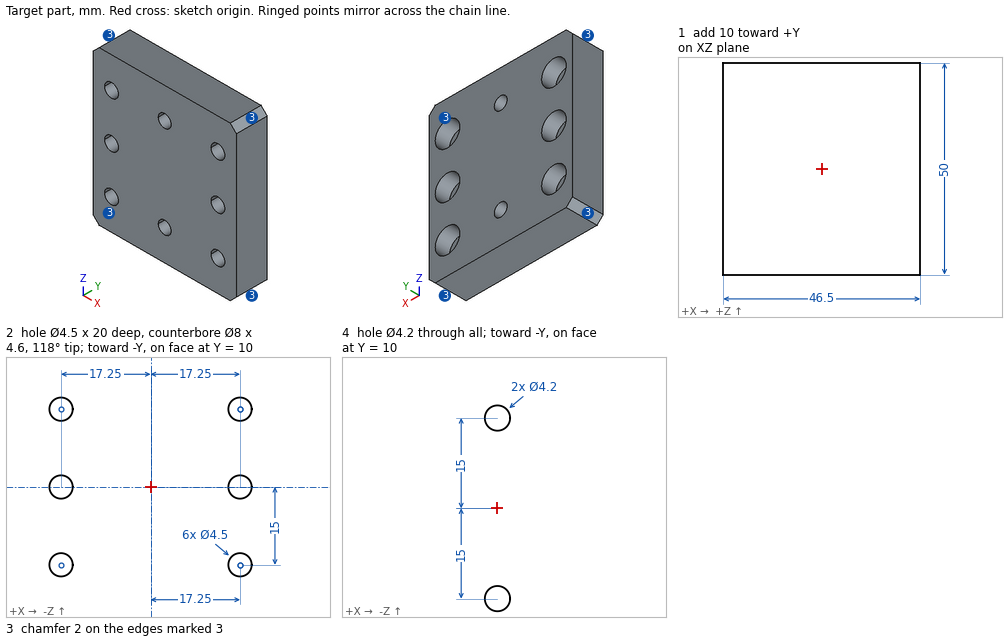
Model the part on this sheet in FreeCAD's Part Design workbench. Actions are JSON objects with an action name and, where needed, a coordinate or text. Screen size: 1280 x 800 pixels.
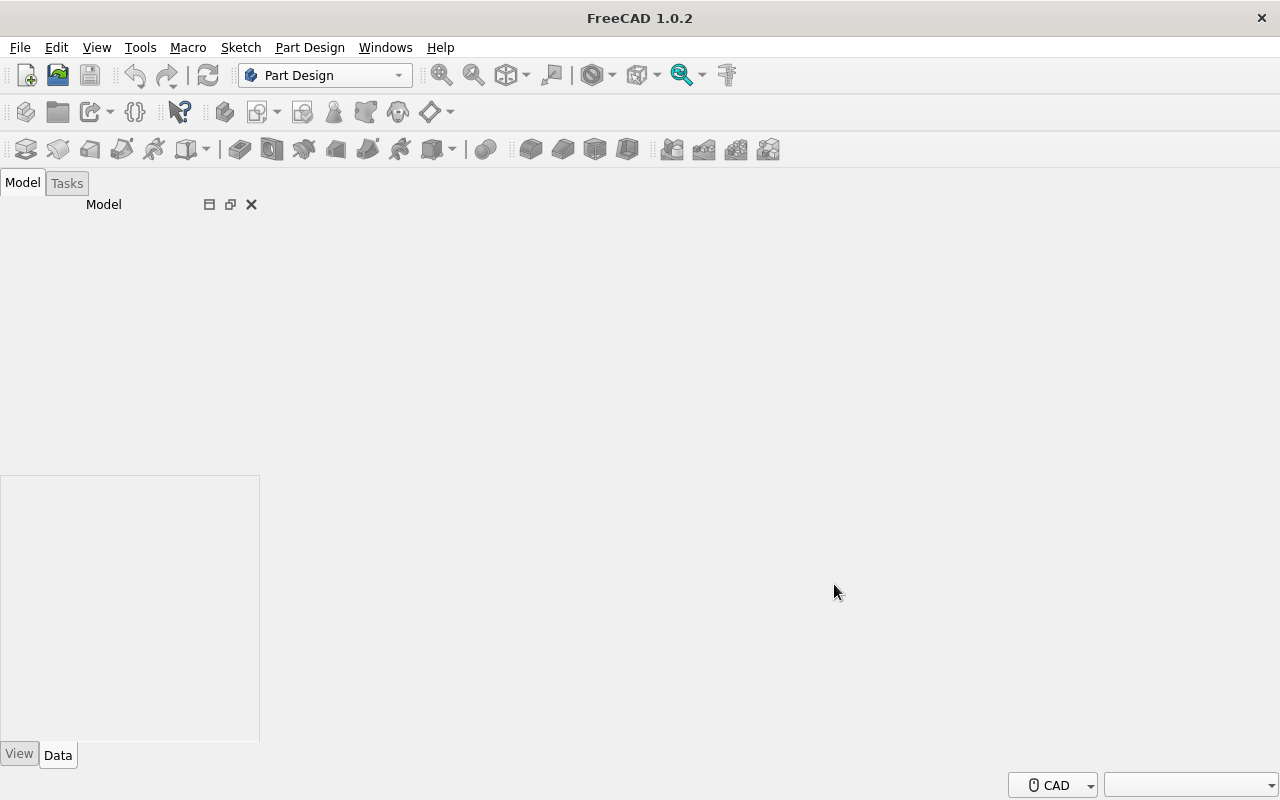
{"action": "key", "text": "ctrl+n"}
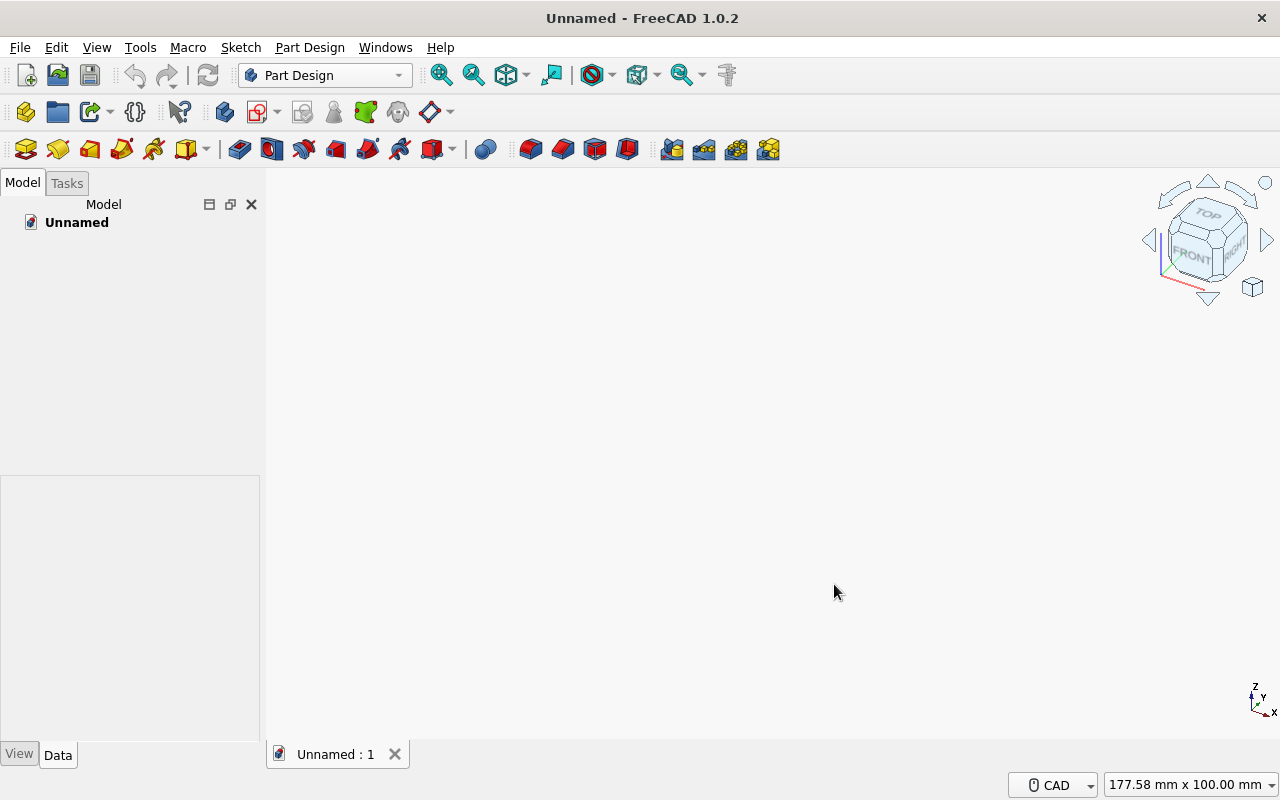
{"action": "left_click", "coordinate": [258, 112]}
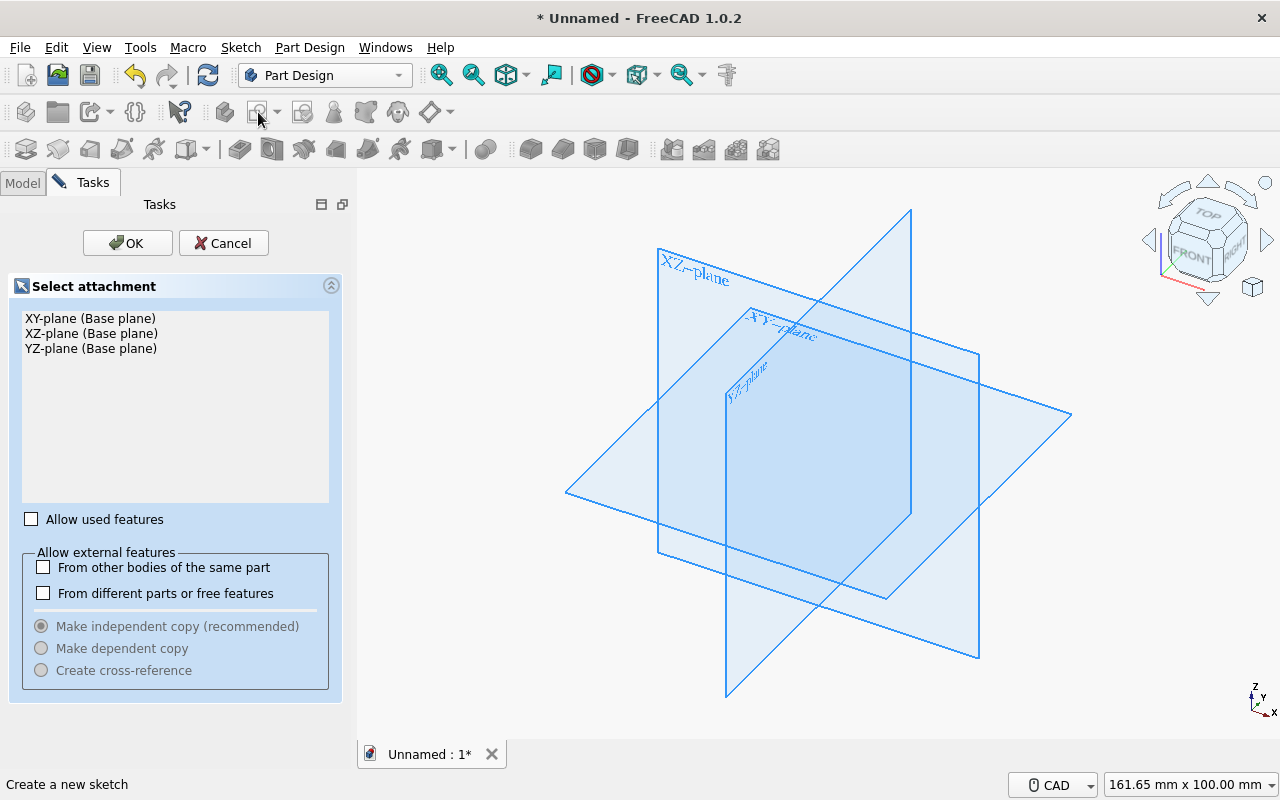
{"action": "left_click", "coordinate": [82, 334]}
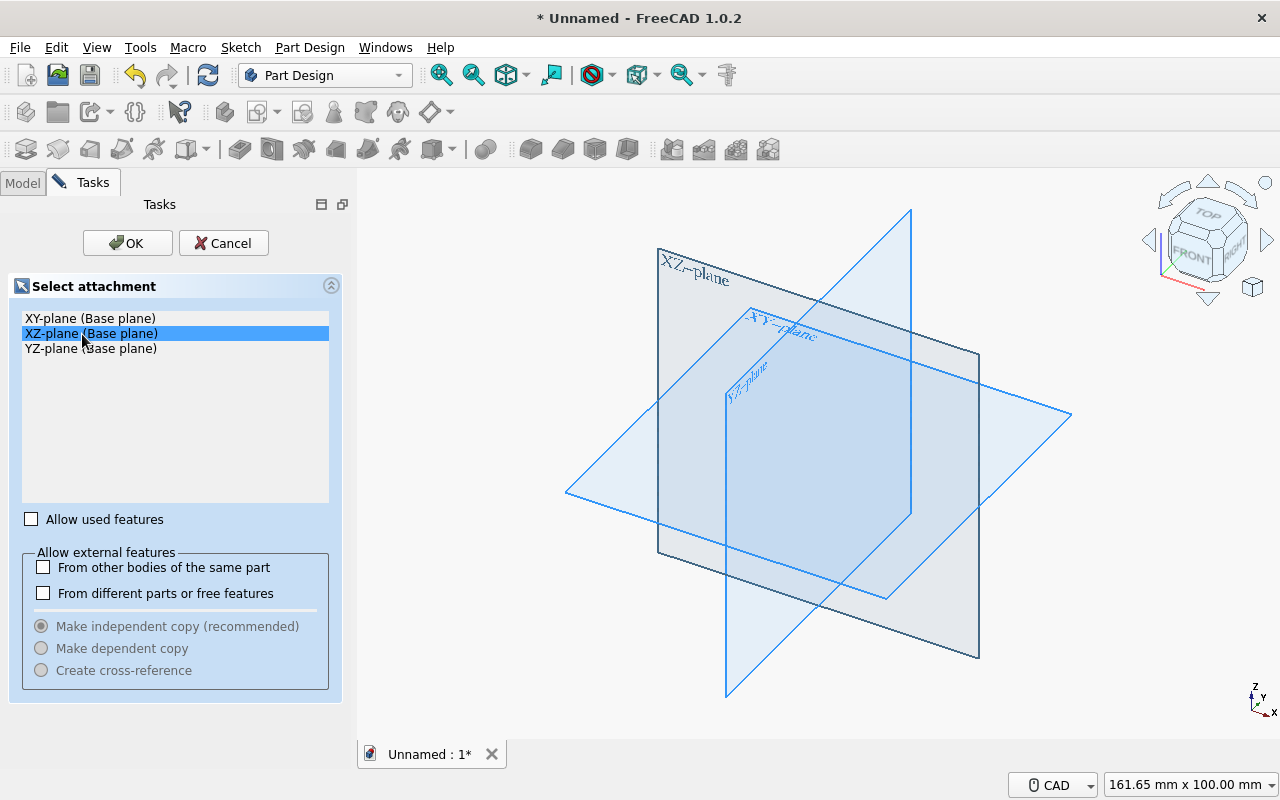
{"action": "left_click", "coordinate": [128, 243]}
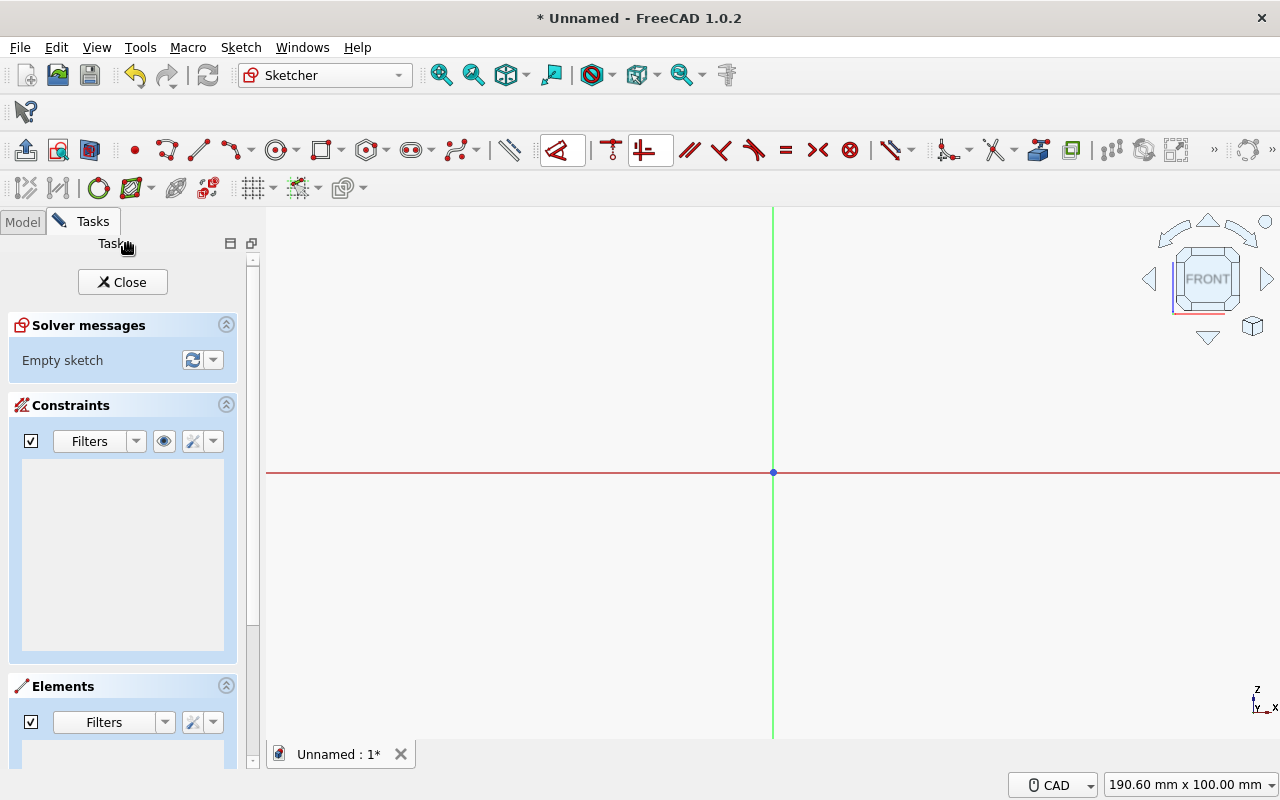
{"action": "left_click", "coordinate": [344, 150]}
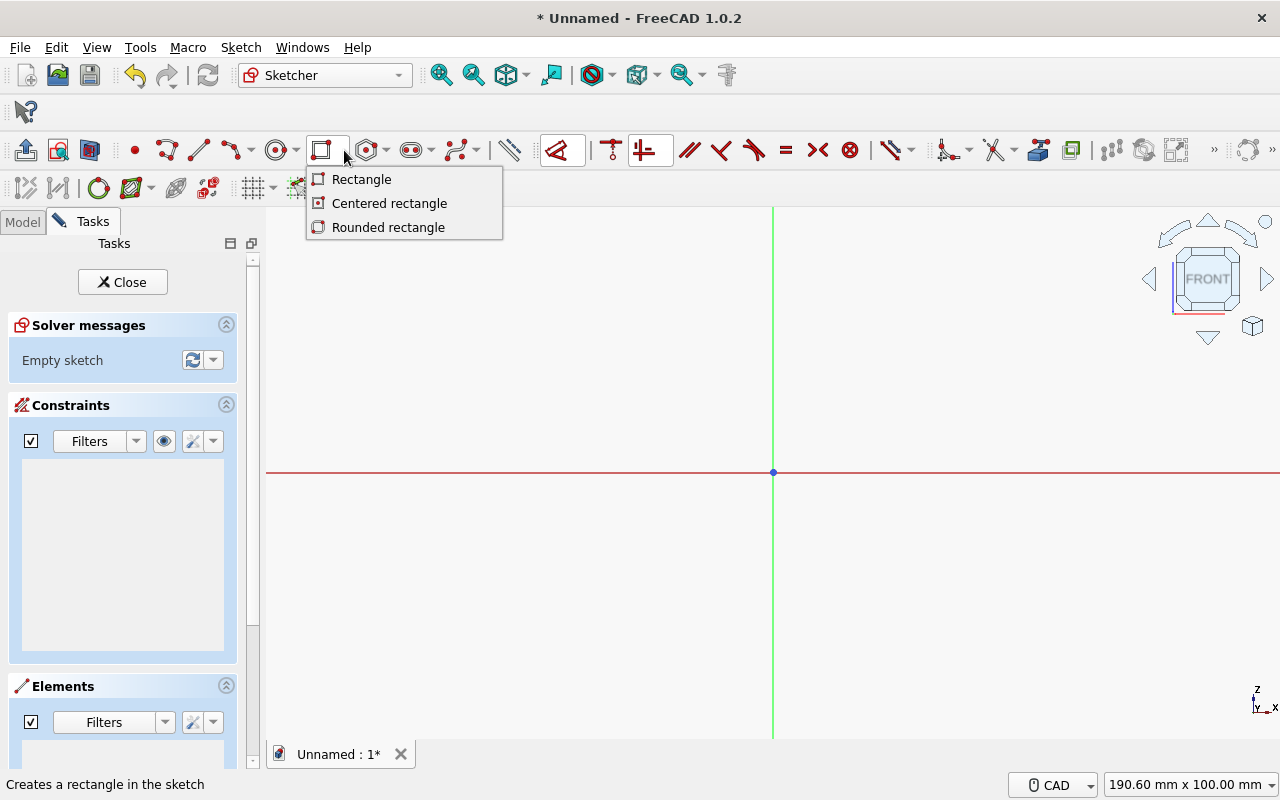
{"action": "left_click", "coordinate": [404, 203]}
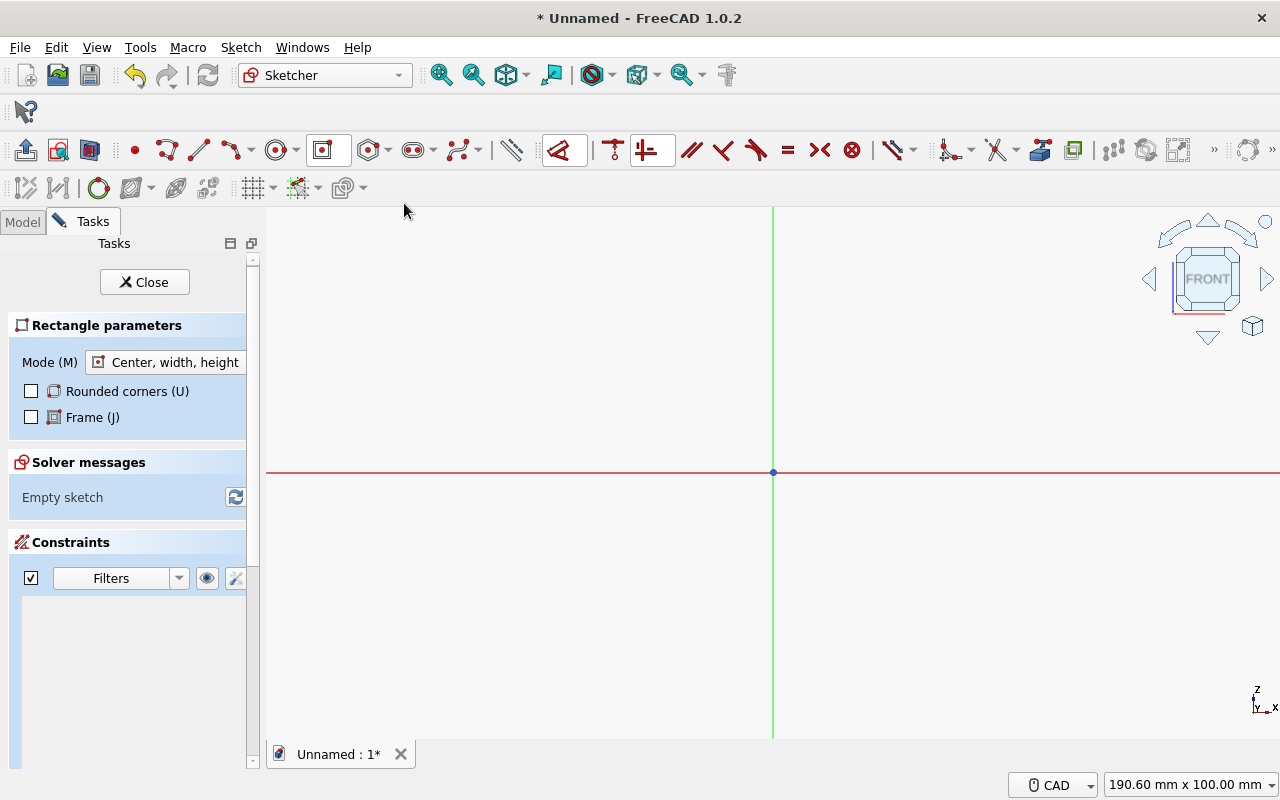
{"action": "left_click", "coordinate": [773, 473]}
{"action": "left_click", "coordinate": [897, 340]}
{"action": "key", "text": "Escape"}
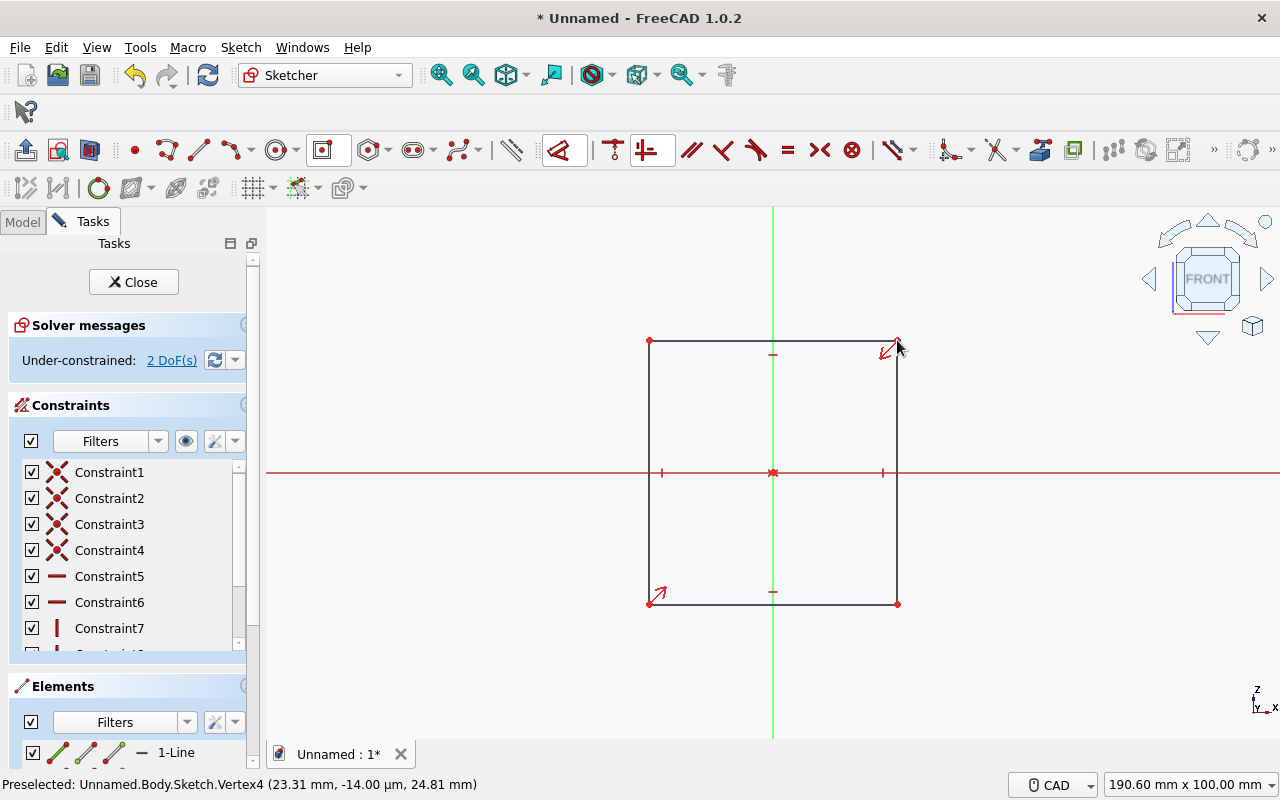
{"action": "left_click", "coordinate": [897, 526]}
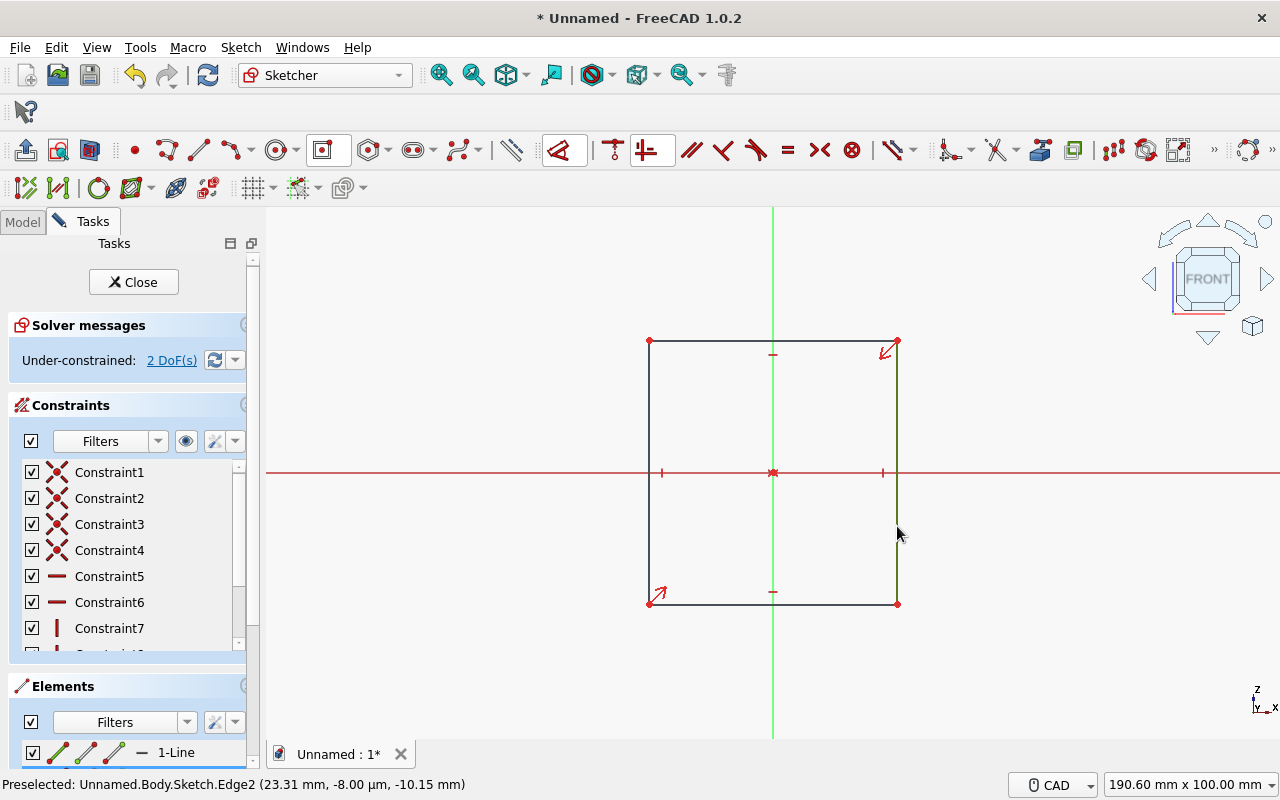
{"action": "key", "text": "i"}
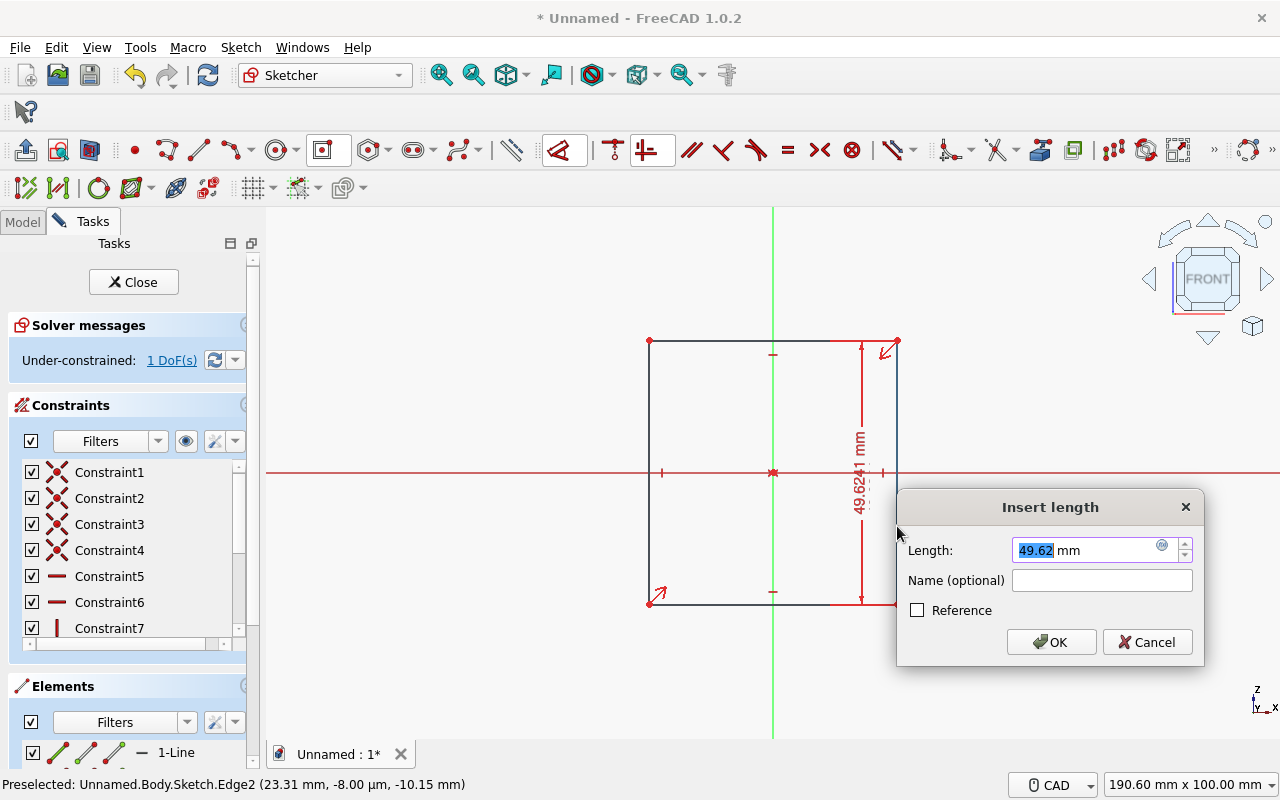
{"action": "type", "text": "50"}
{"action": "key", "text": "Return"}